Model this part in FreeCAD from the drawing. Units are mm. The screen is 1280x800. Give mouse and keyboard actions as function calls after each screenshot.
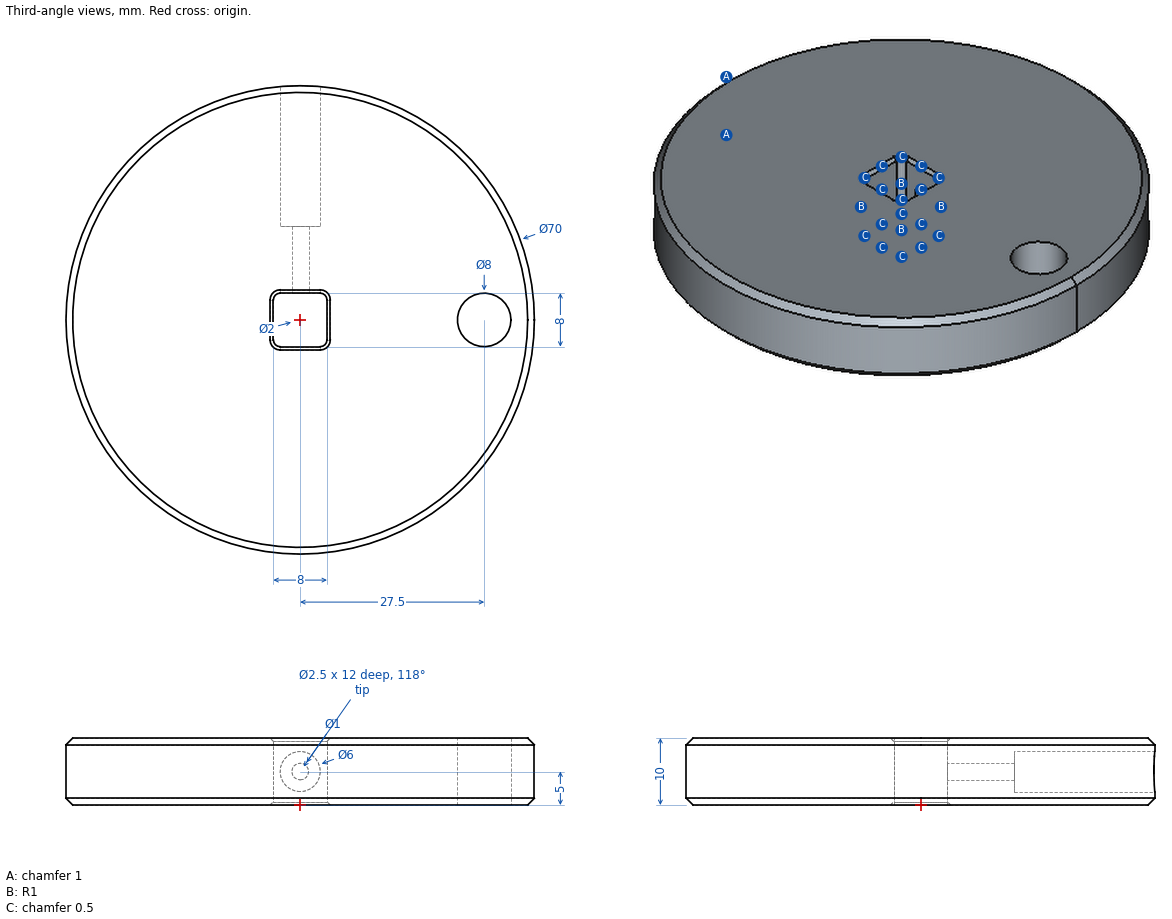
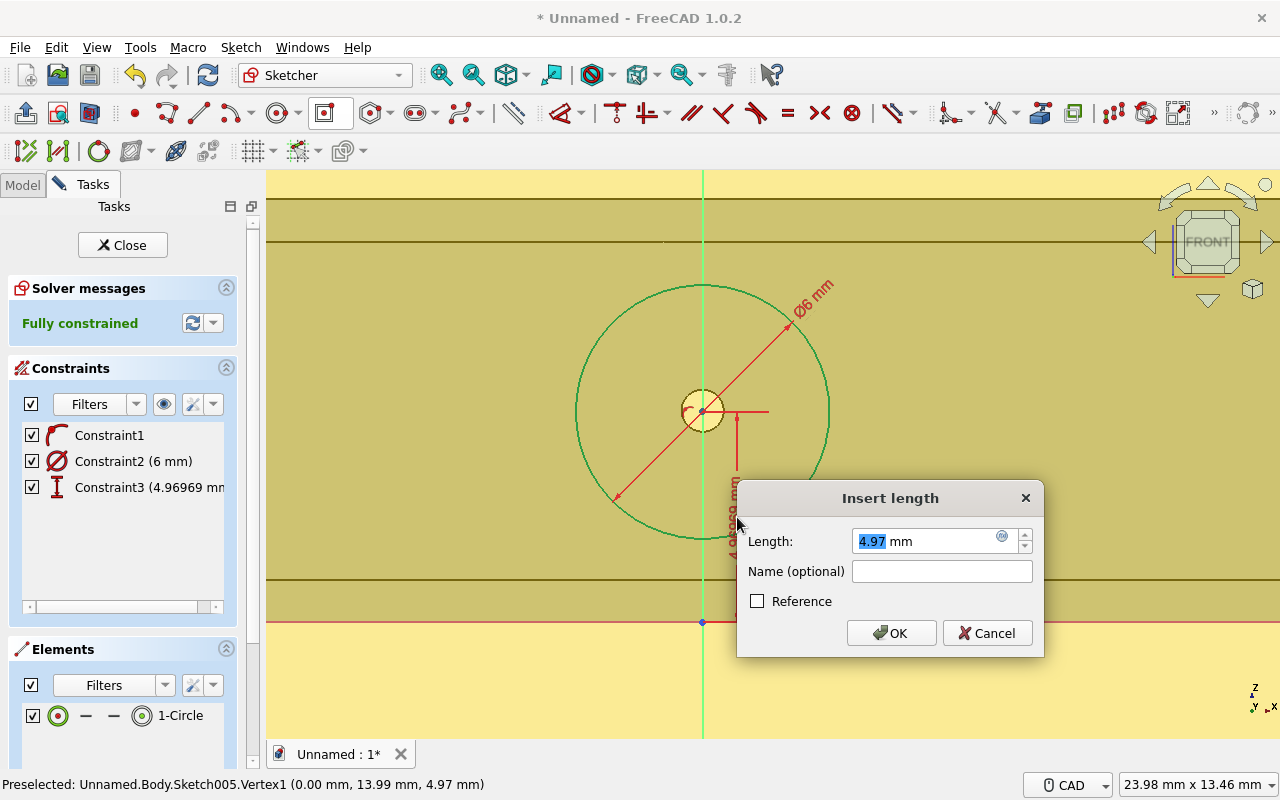
text(5)
key(Return)
key(Escape)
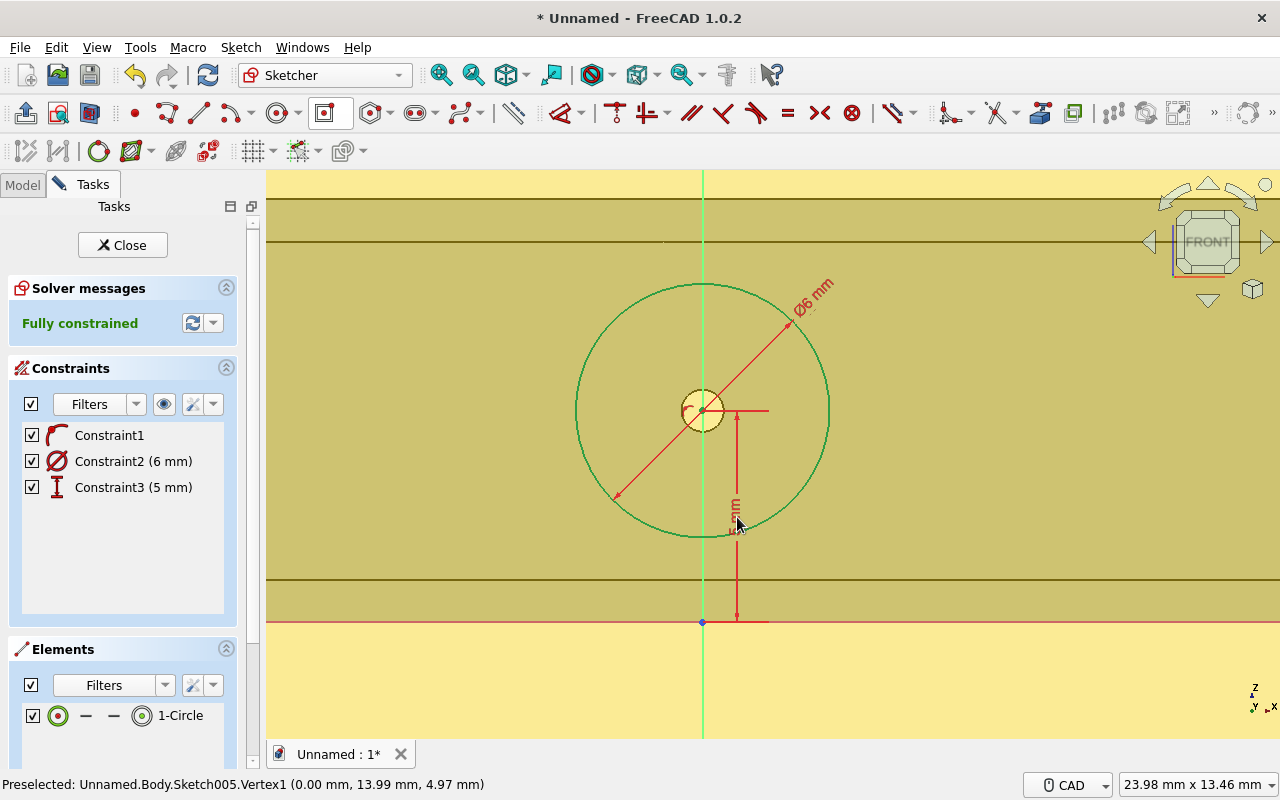
click(123, 245)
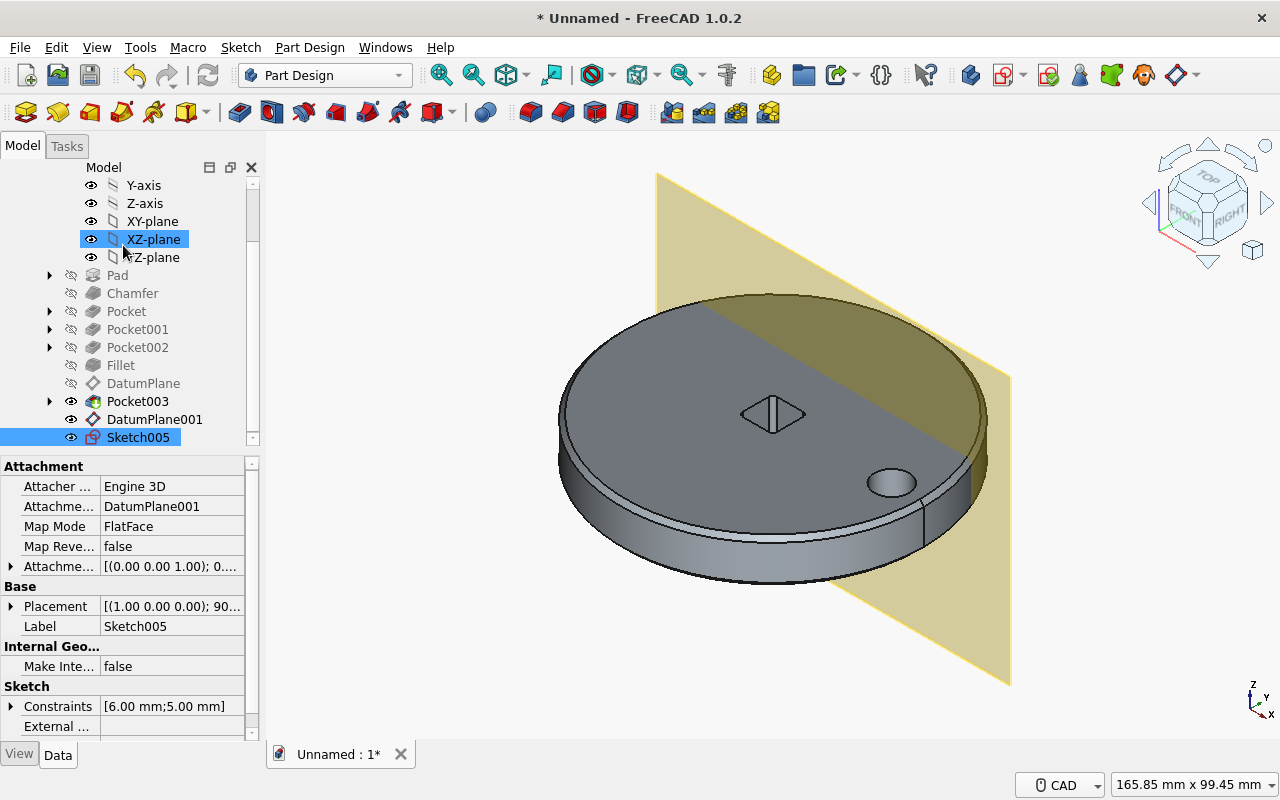
click(240, 112)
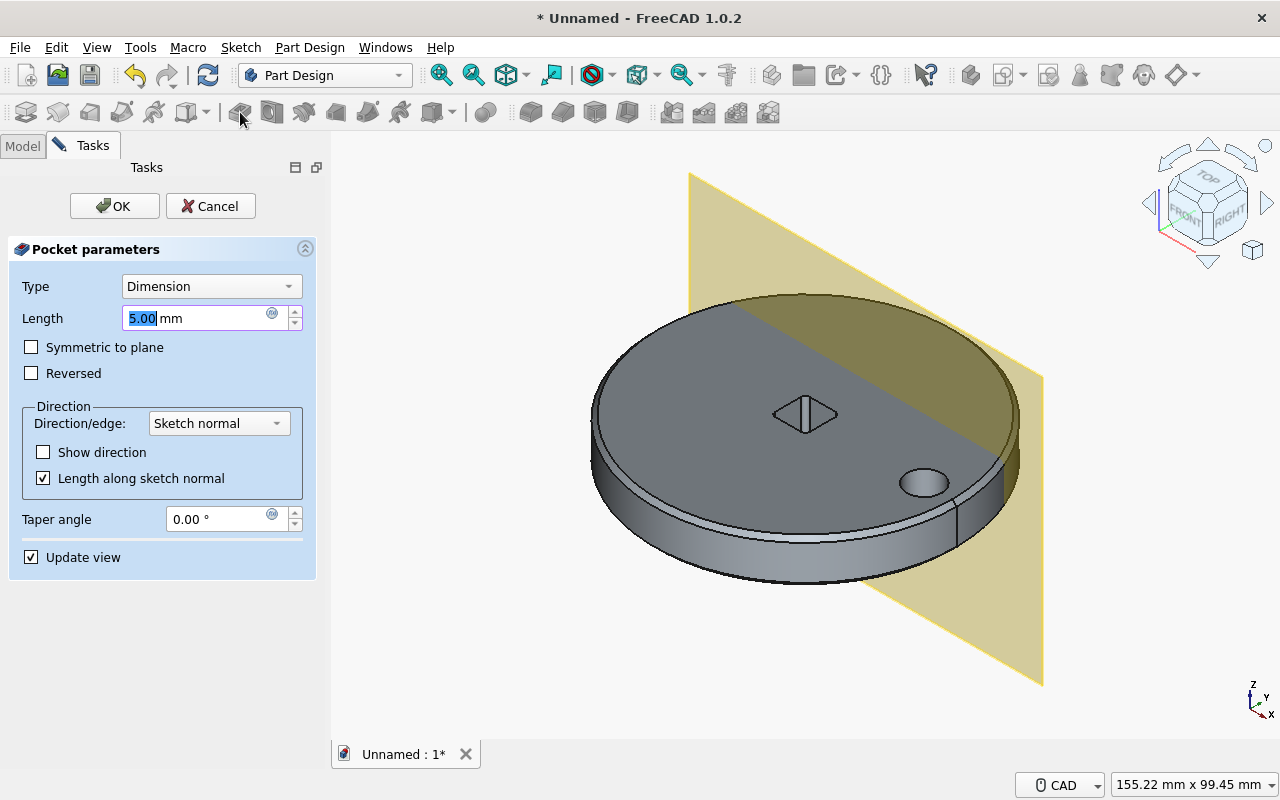
click(212, 286)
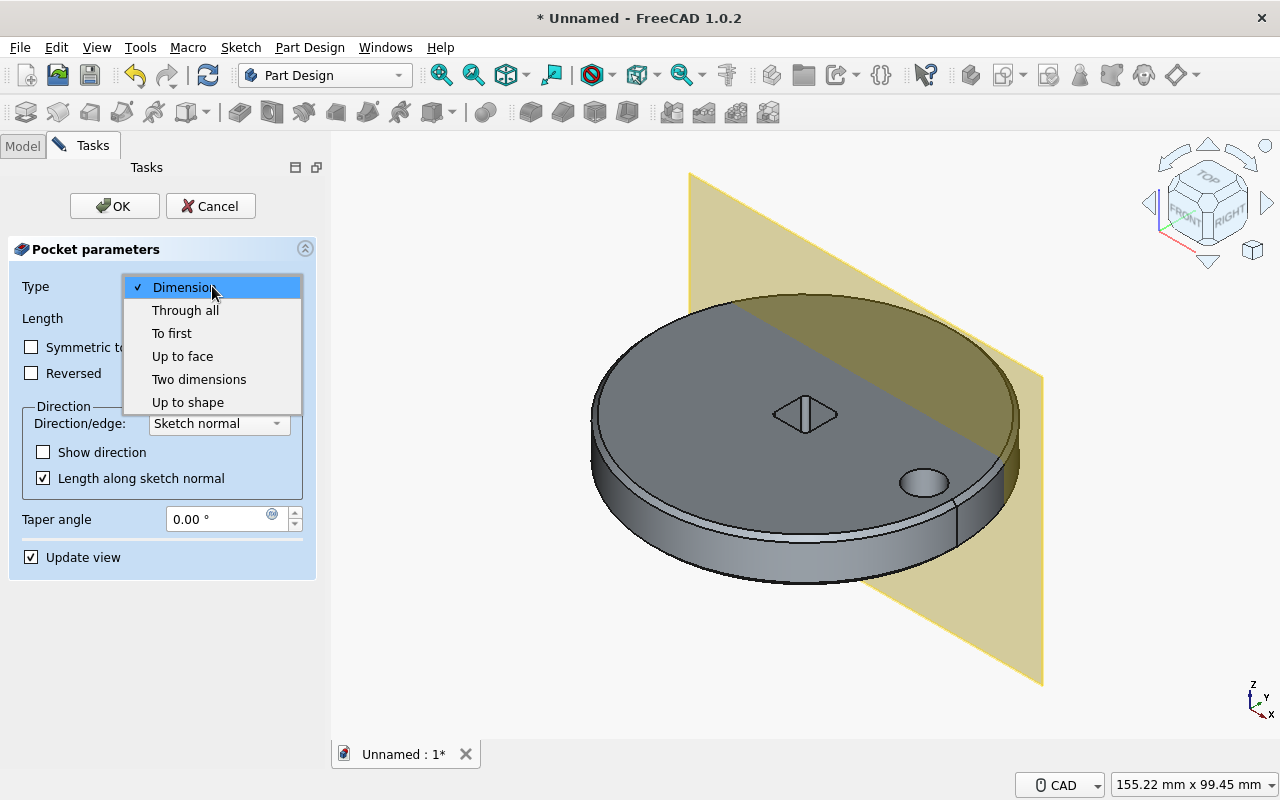
click(212, 310)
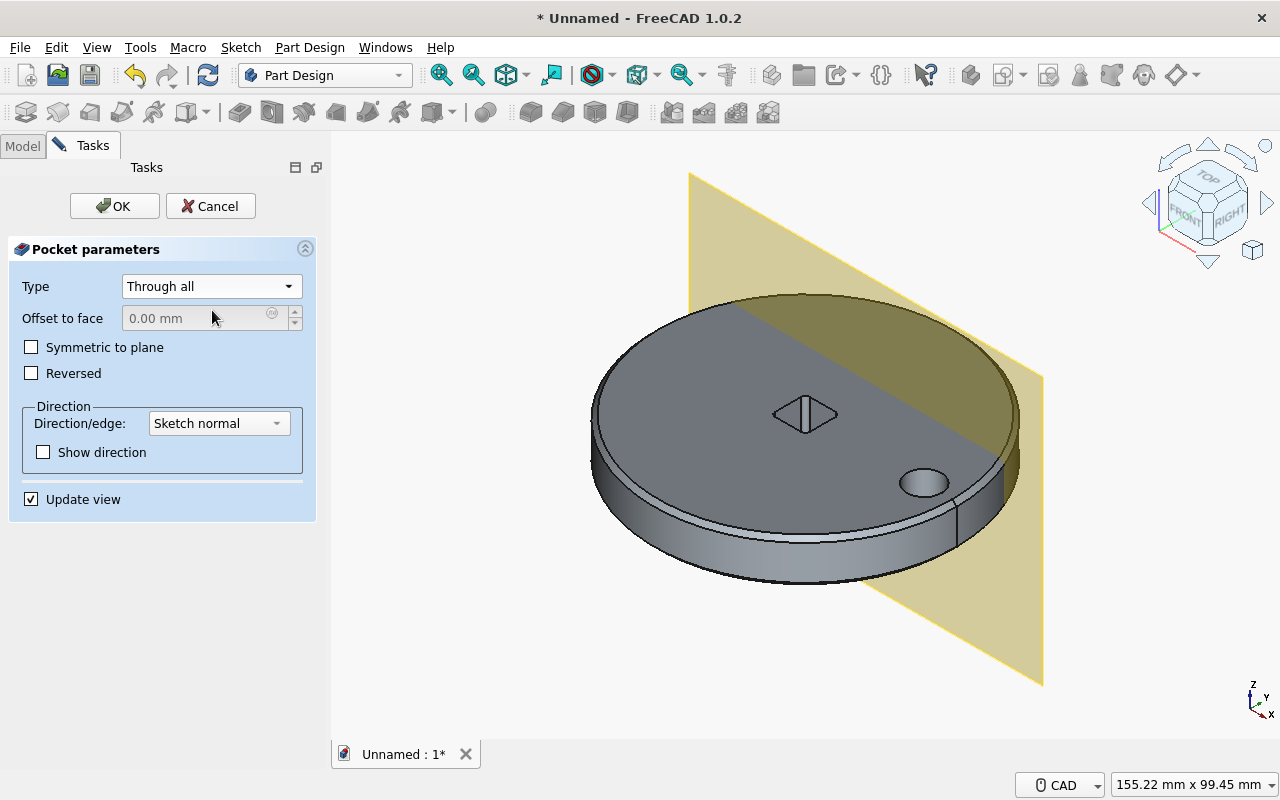
click(115, 206)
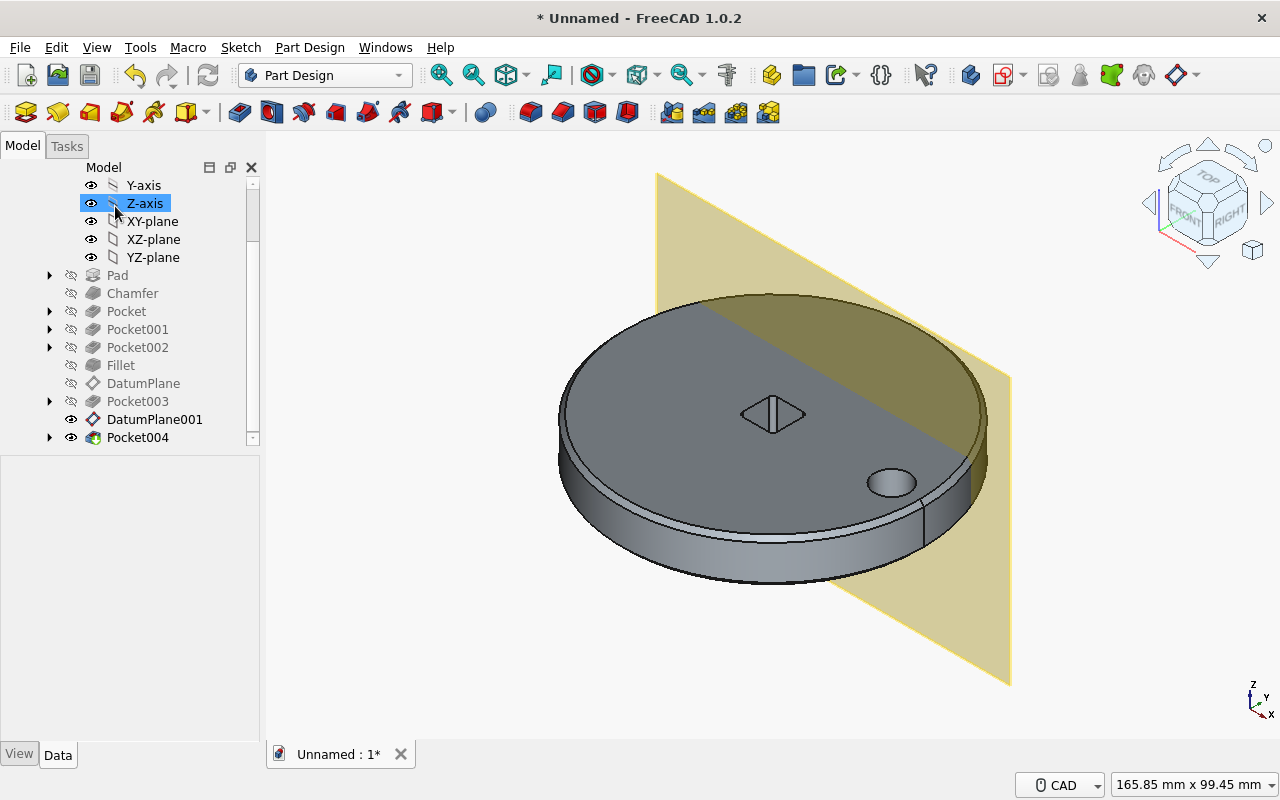
click(116, 419)
key(space)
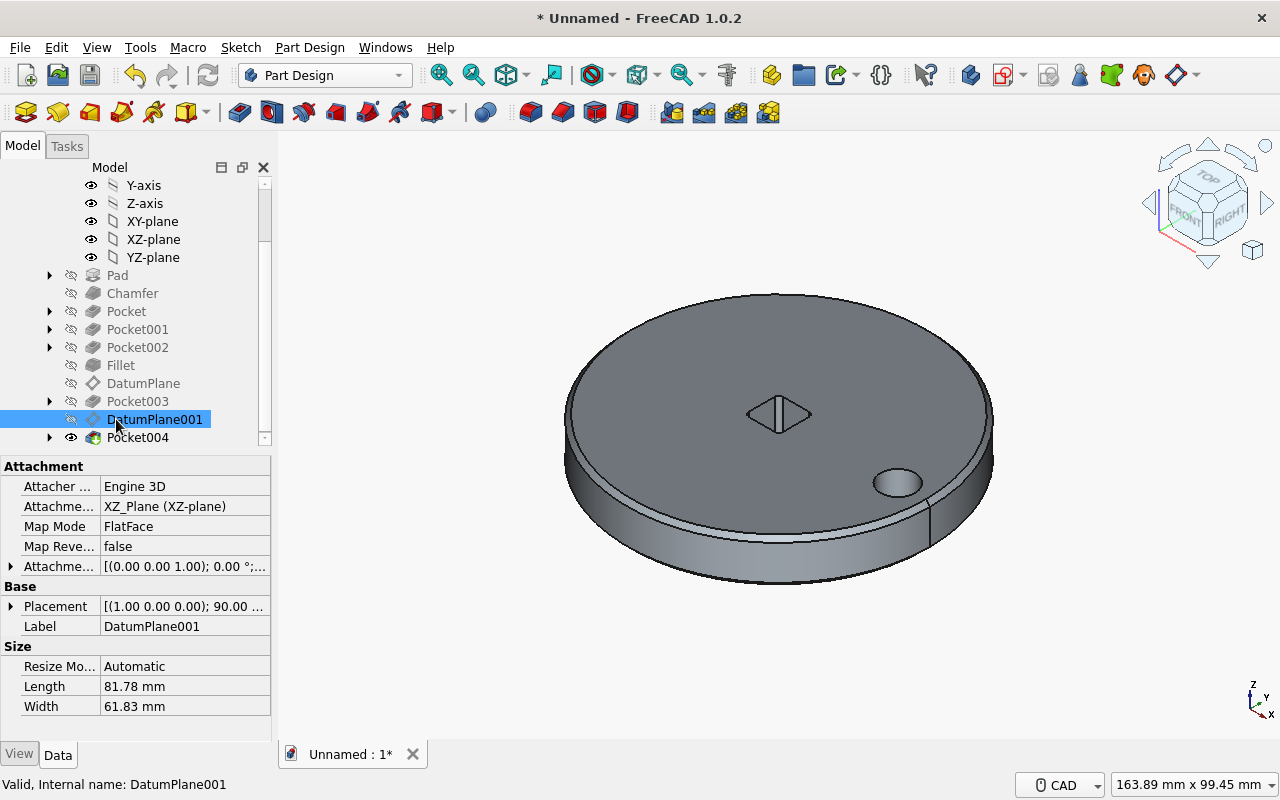
key(4)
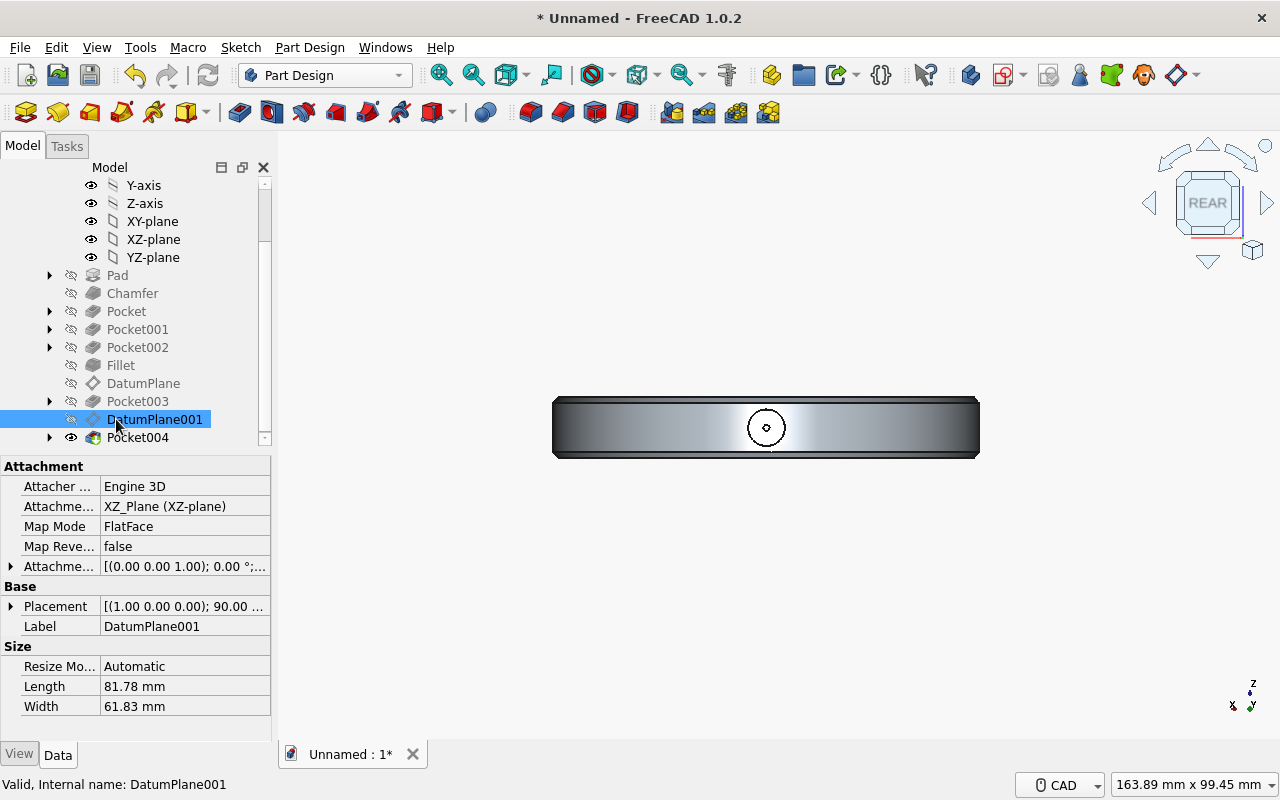
click(442, 76)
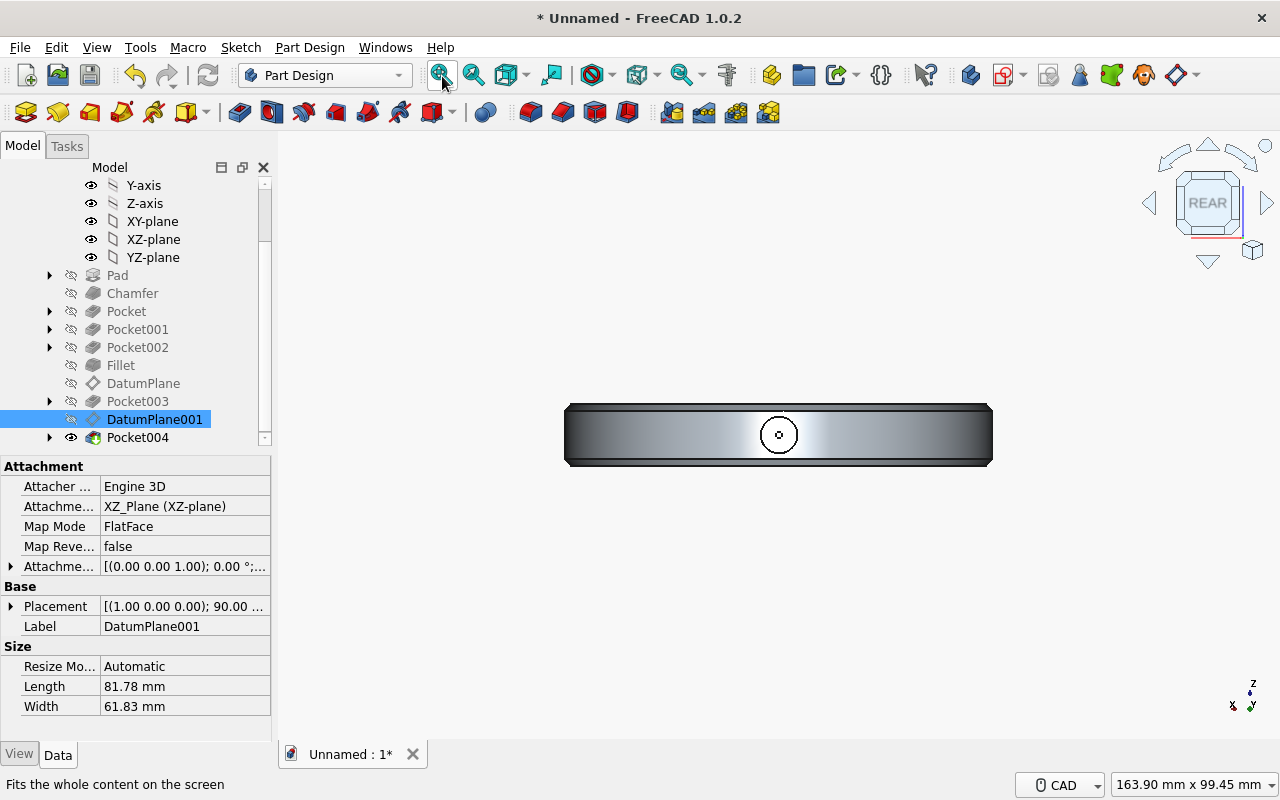
key(5)